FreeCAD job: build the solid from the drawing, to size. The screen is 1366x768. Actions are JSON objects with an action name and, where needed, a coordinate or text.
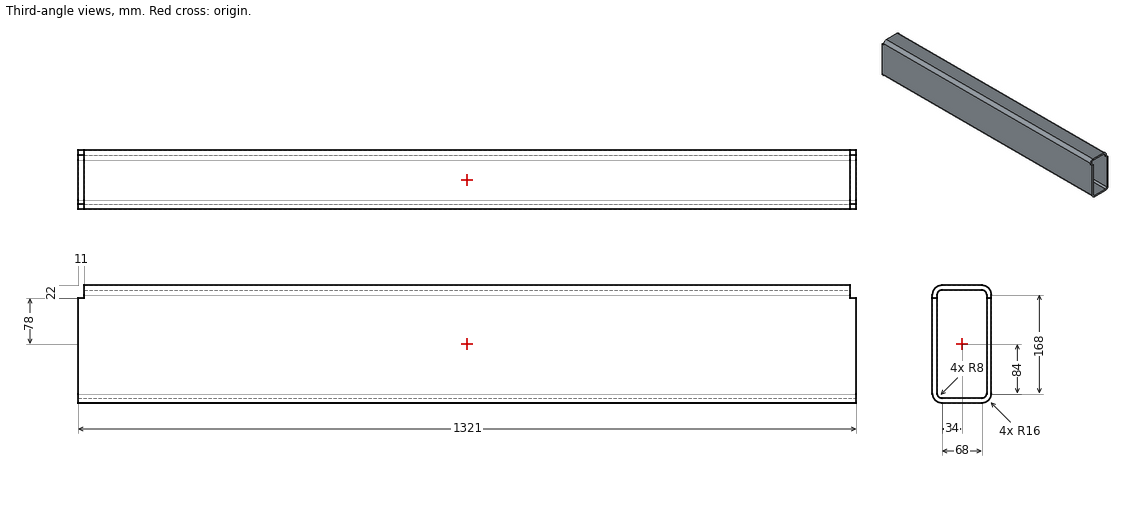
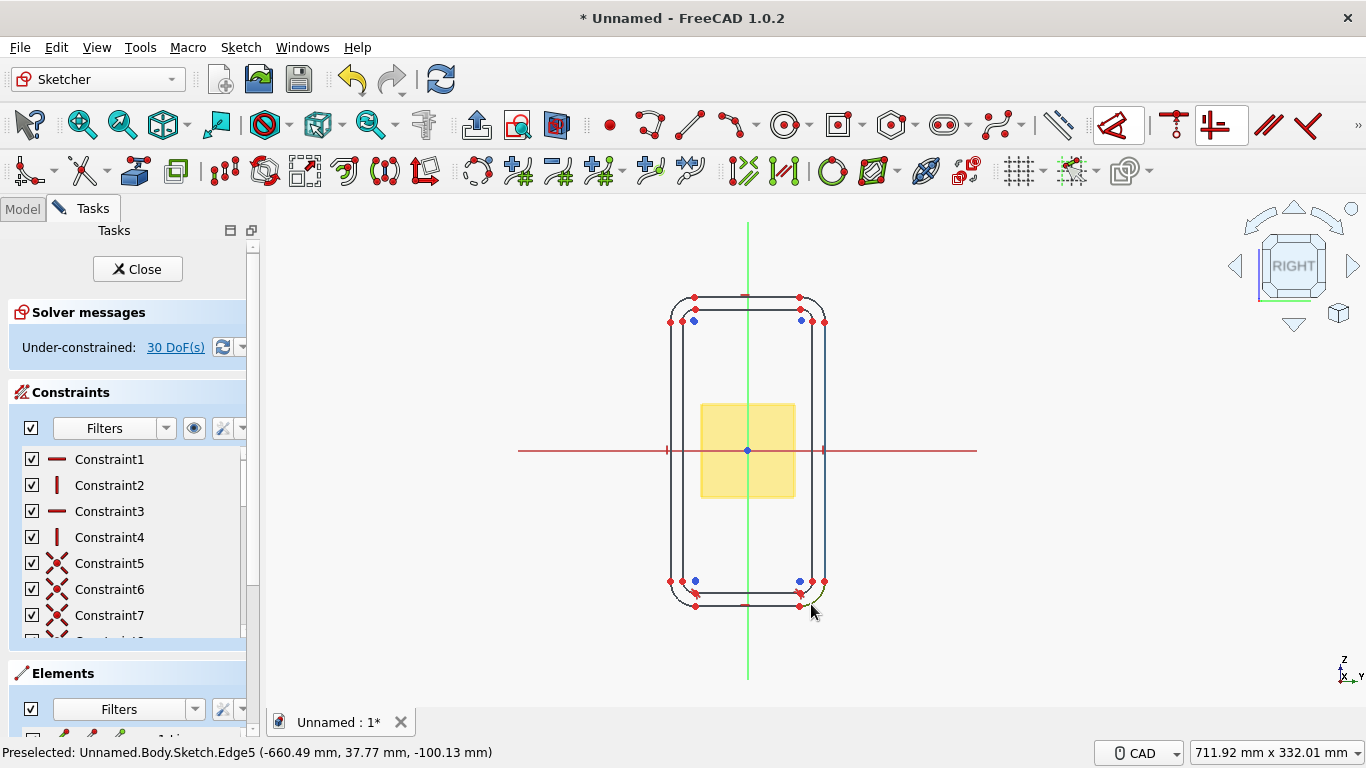
{"action": "key", "text": "t"}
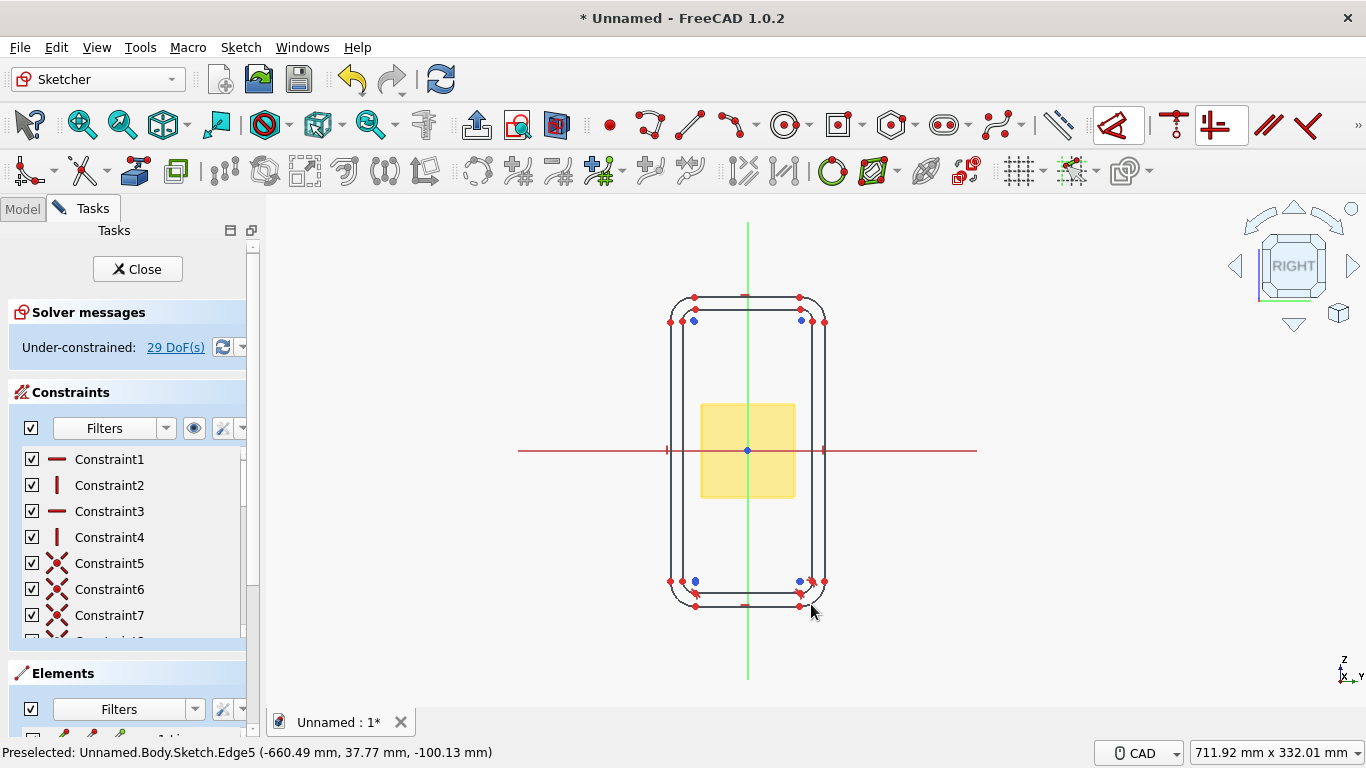
{"action": "left_click", "coordinate": [825, 504]}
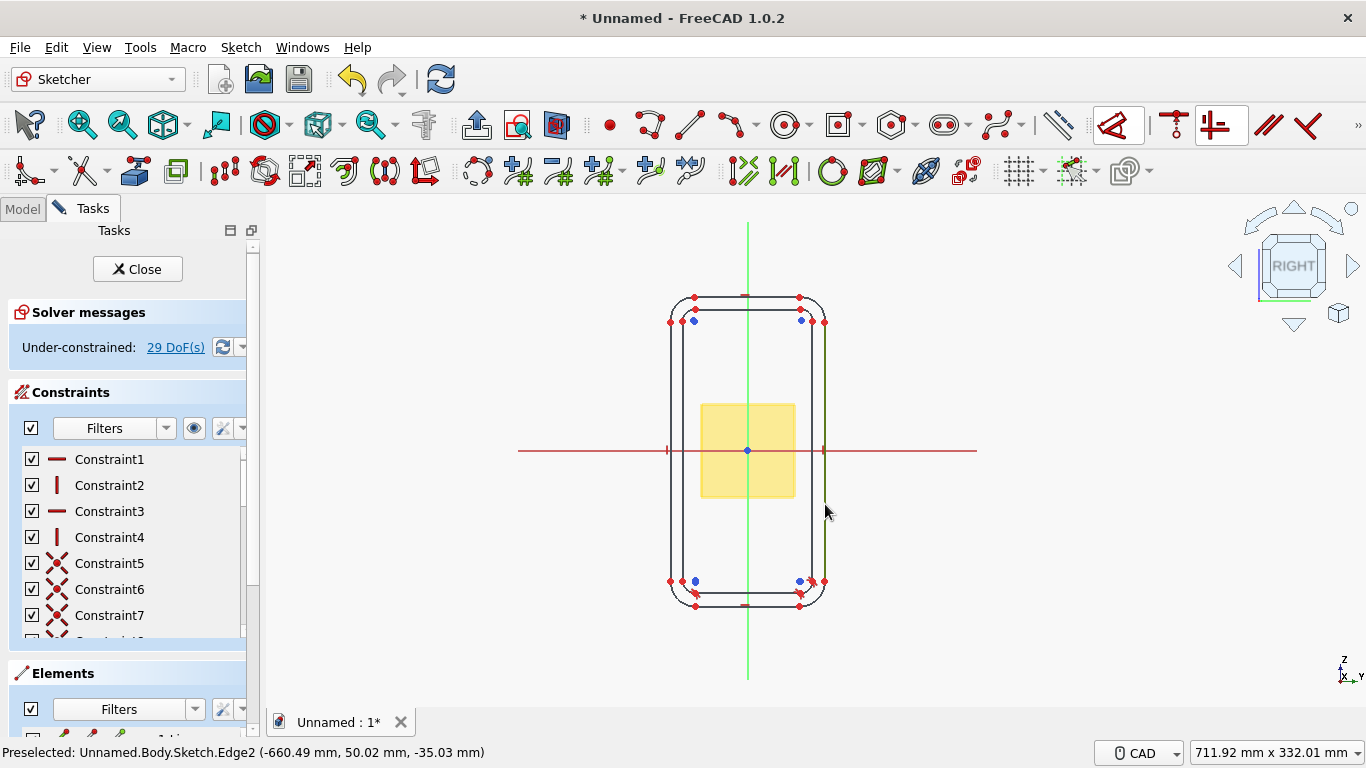
{"action": "left_click", "coordinate": [823, 311]}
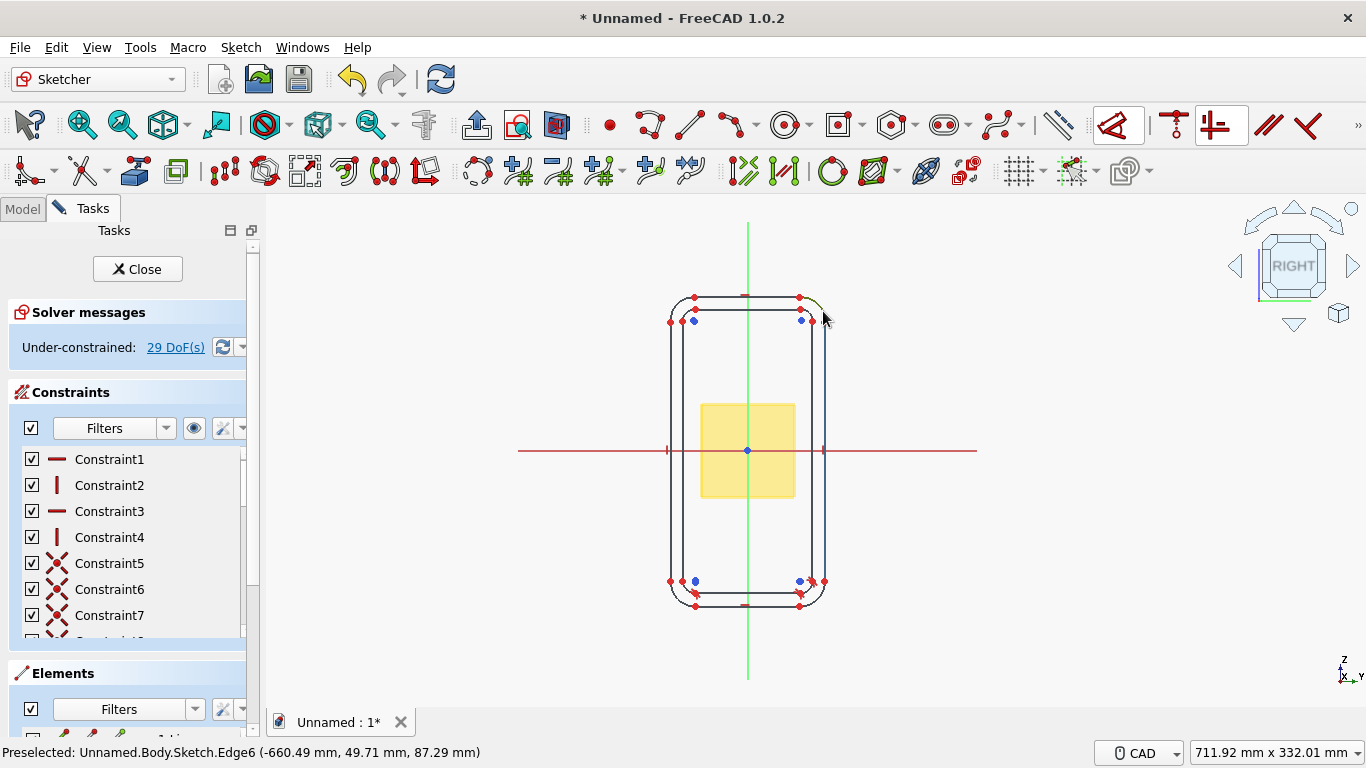
{"action": "key", "text": "t"}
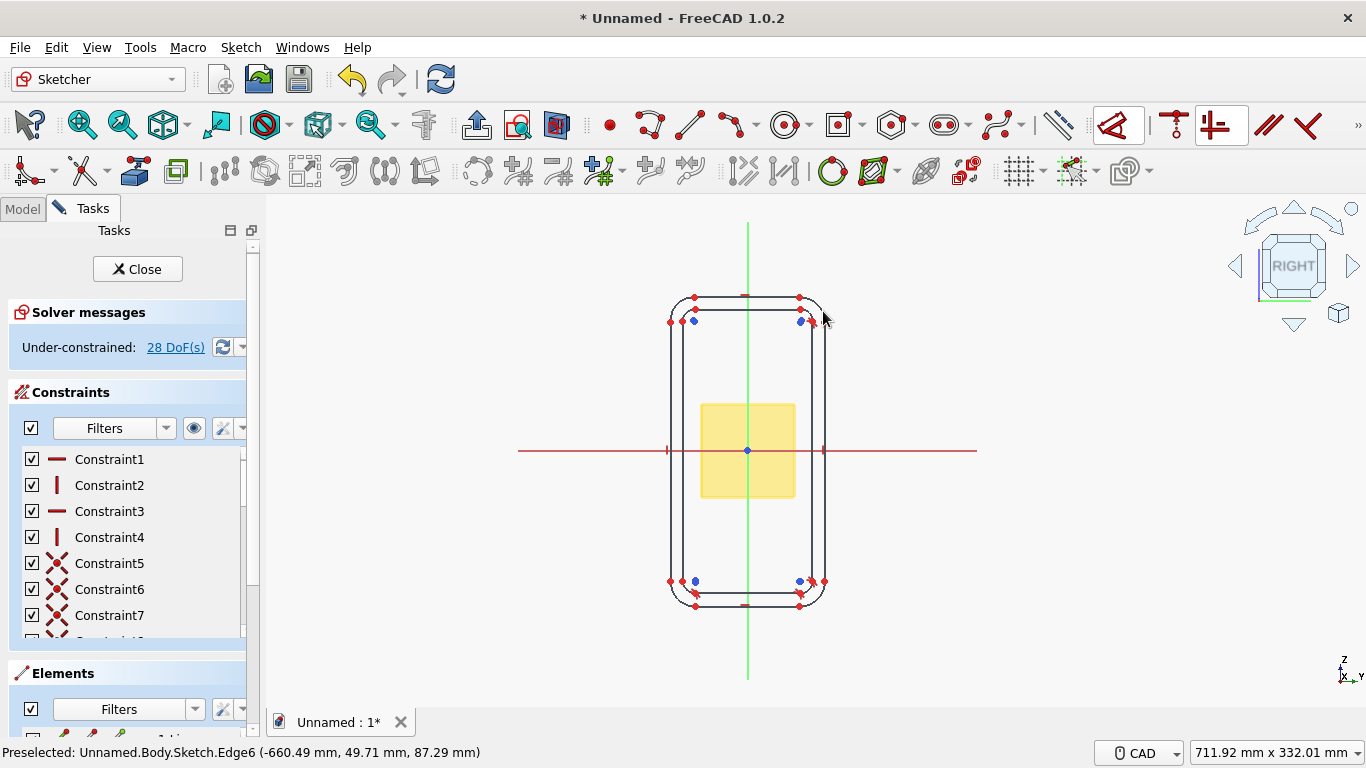
{"action": "left_click", "coordinate": [768, 297]}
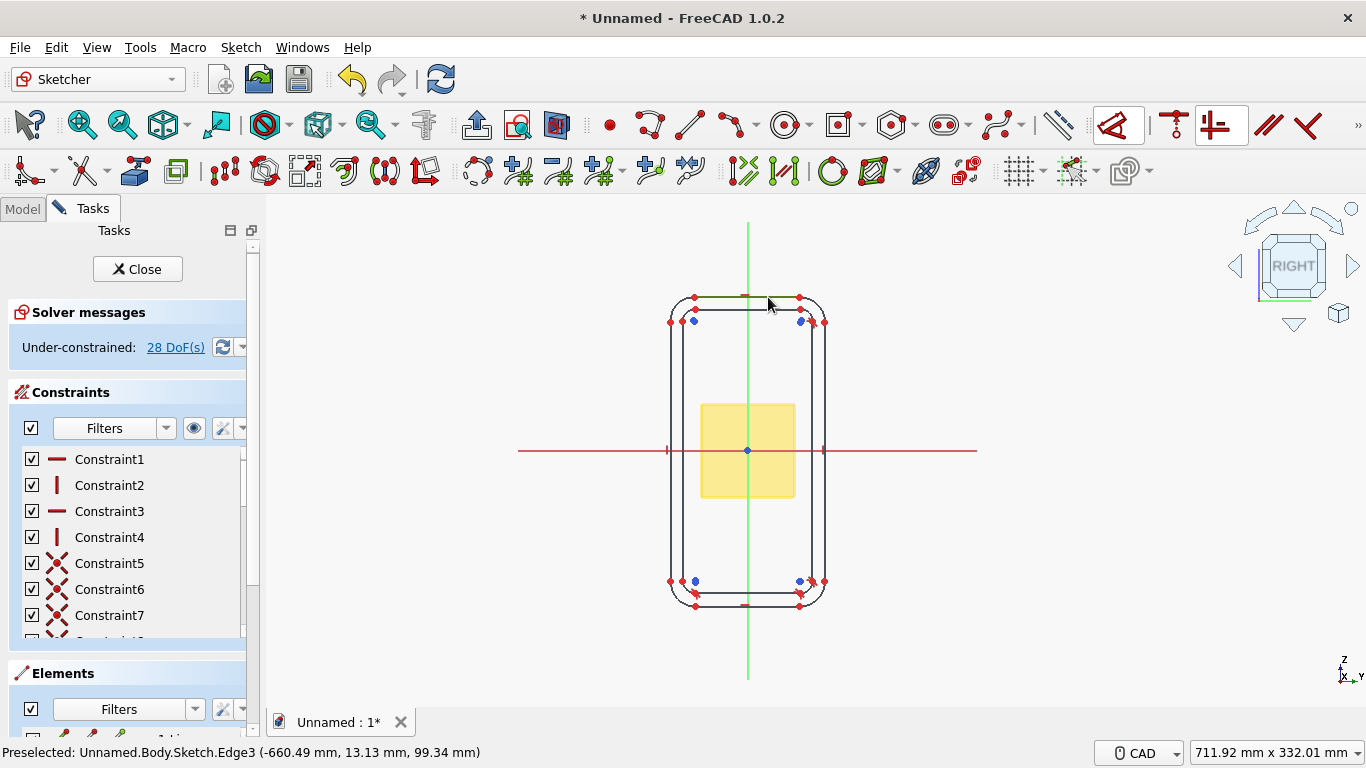
{"action": "left_click", "coordinate": [822, 311]}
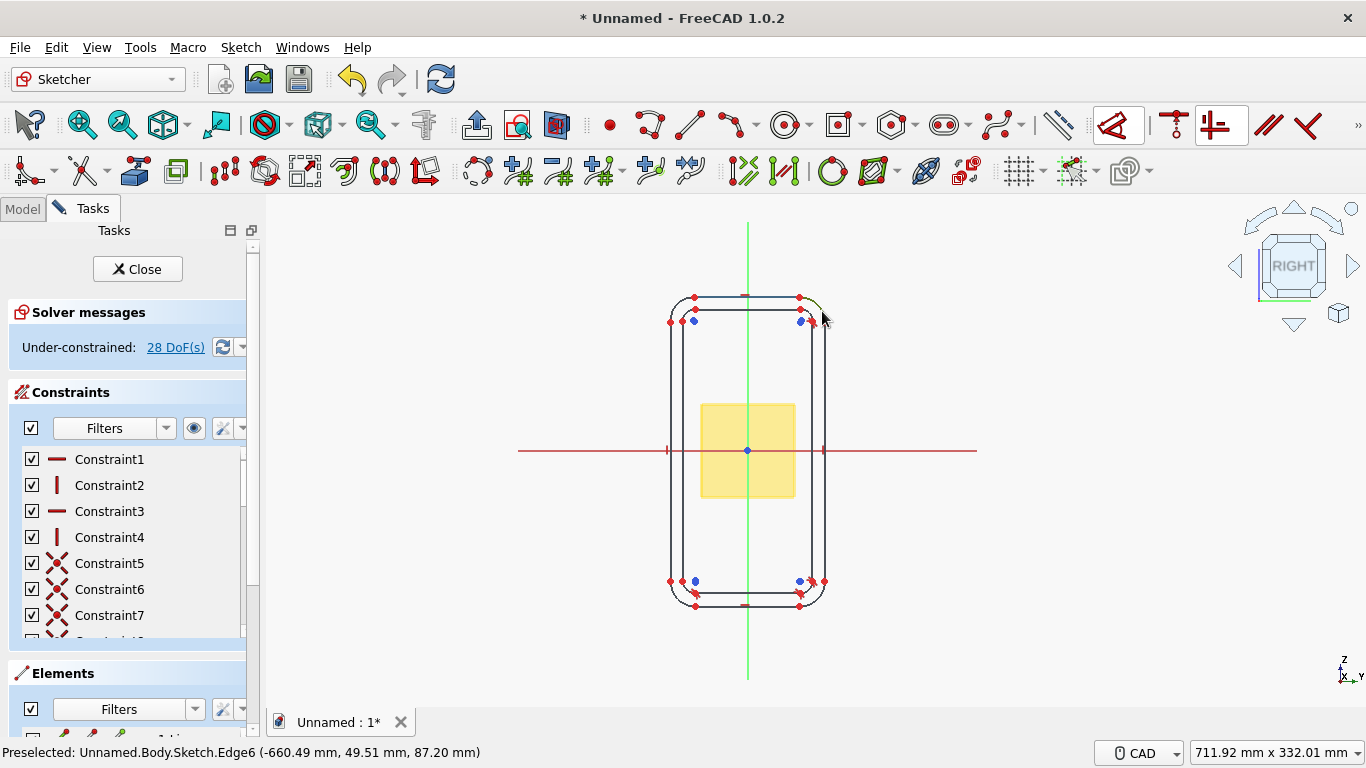
{"action": "key", "text": "t"}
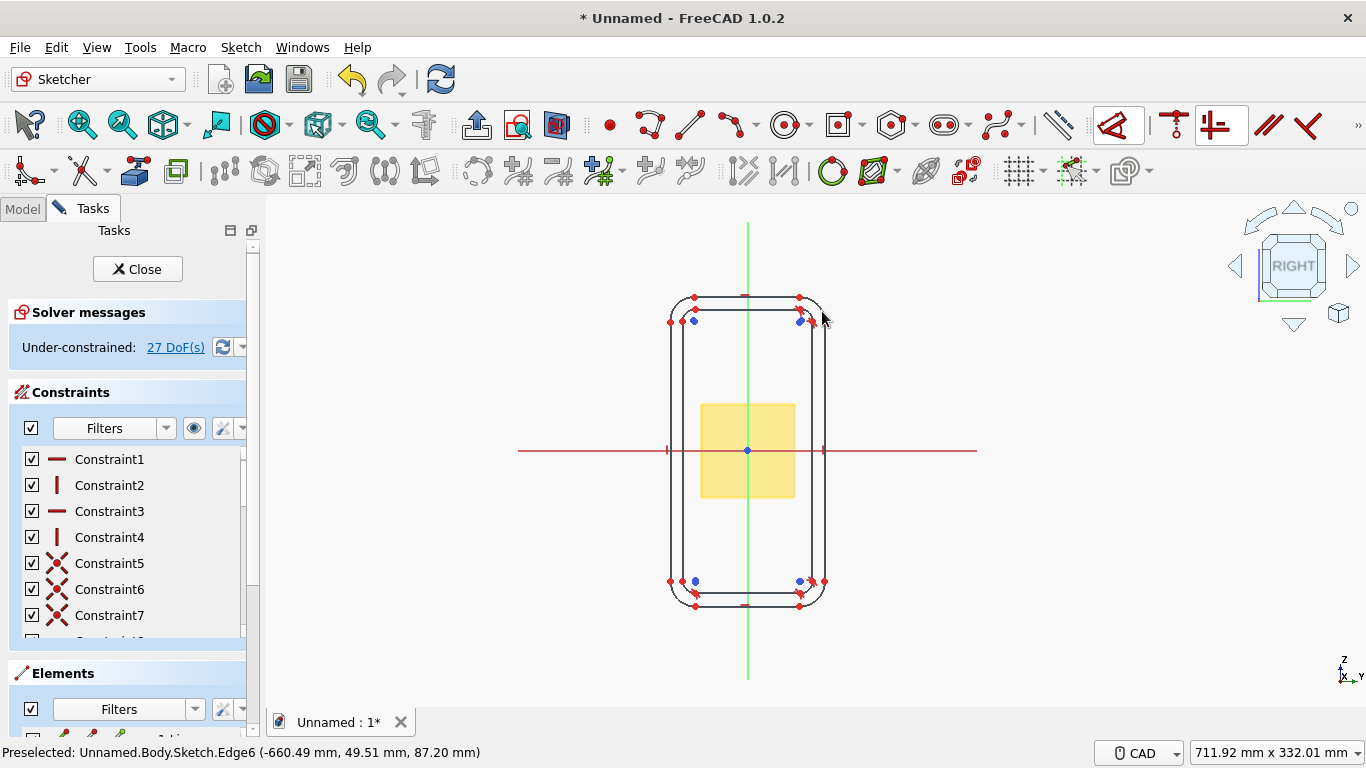
{"action": "left_click", "coordinate": [768, 297]}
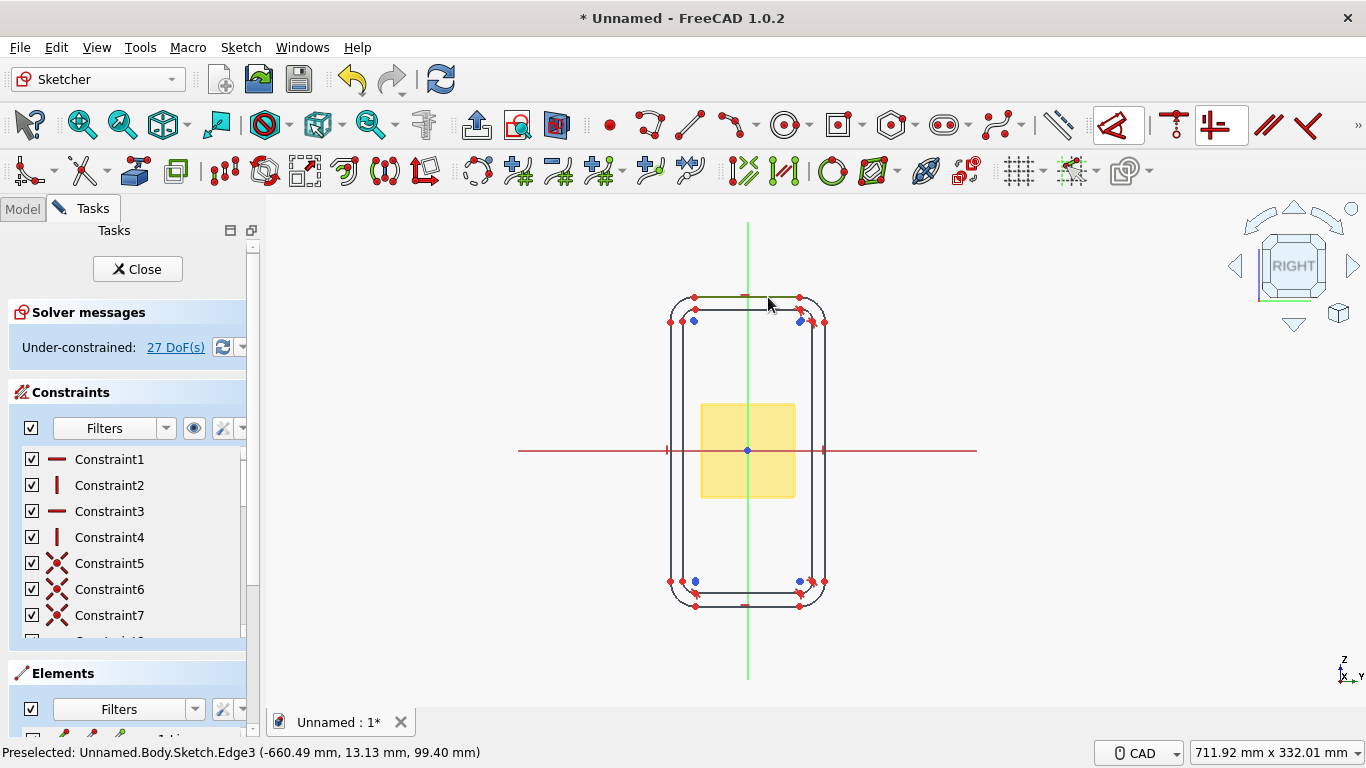
{"action": "left_click", "coordinate": [683, 300]}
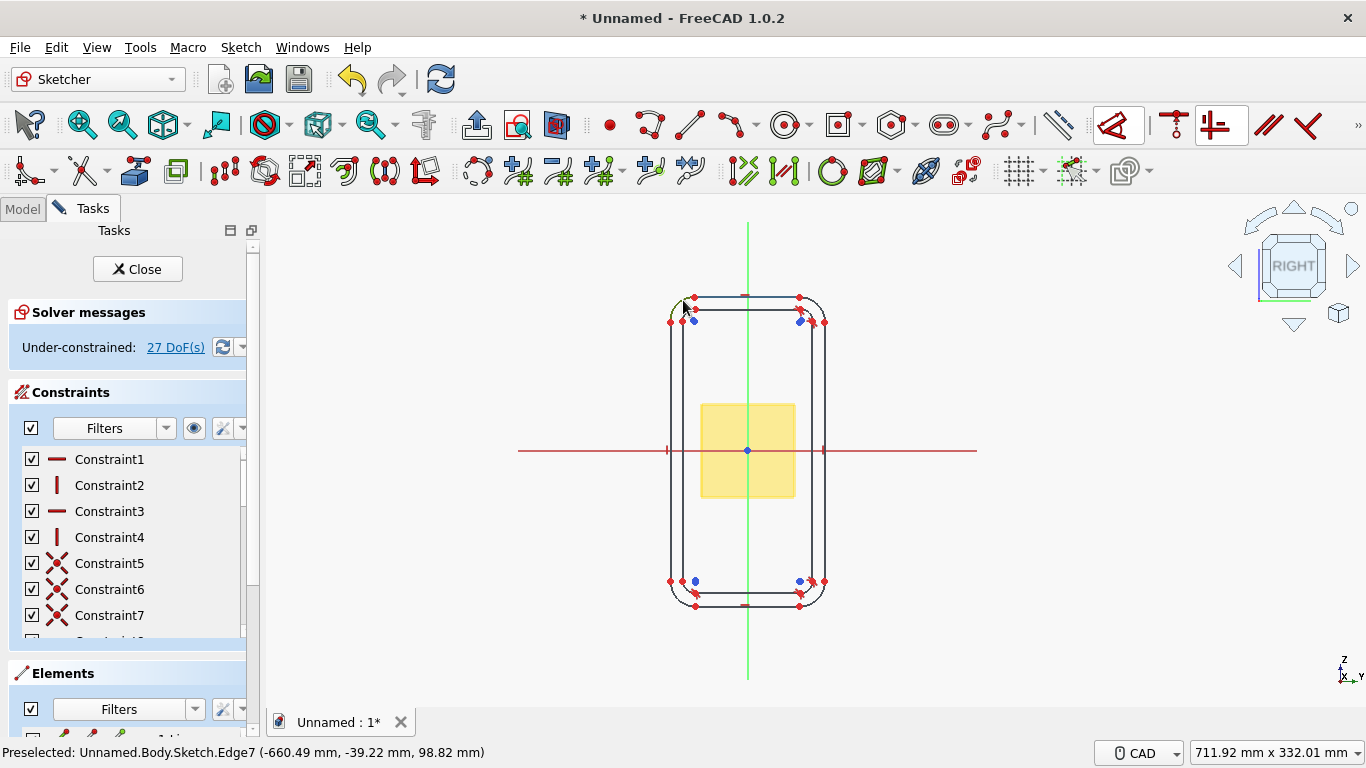
{"action": "key", "text": "t"}